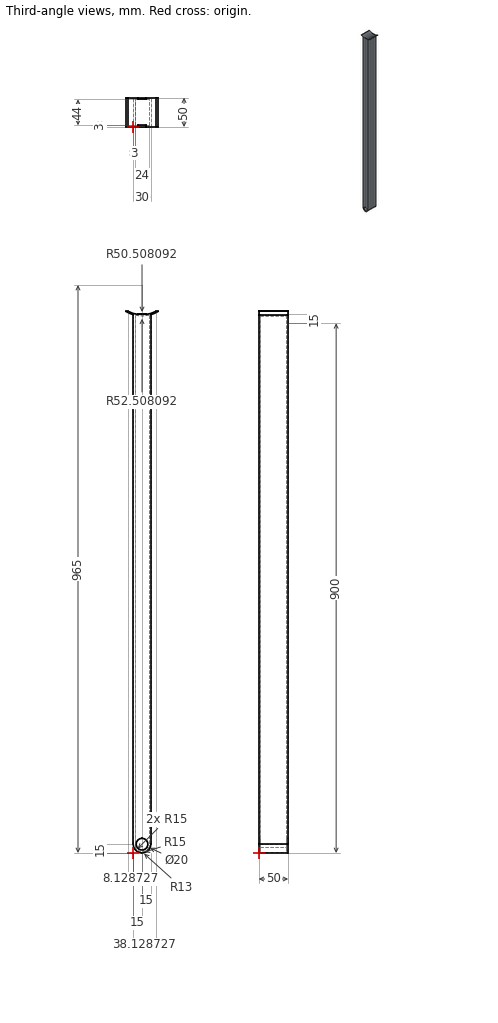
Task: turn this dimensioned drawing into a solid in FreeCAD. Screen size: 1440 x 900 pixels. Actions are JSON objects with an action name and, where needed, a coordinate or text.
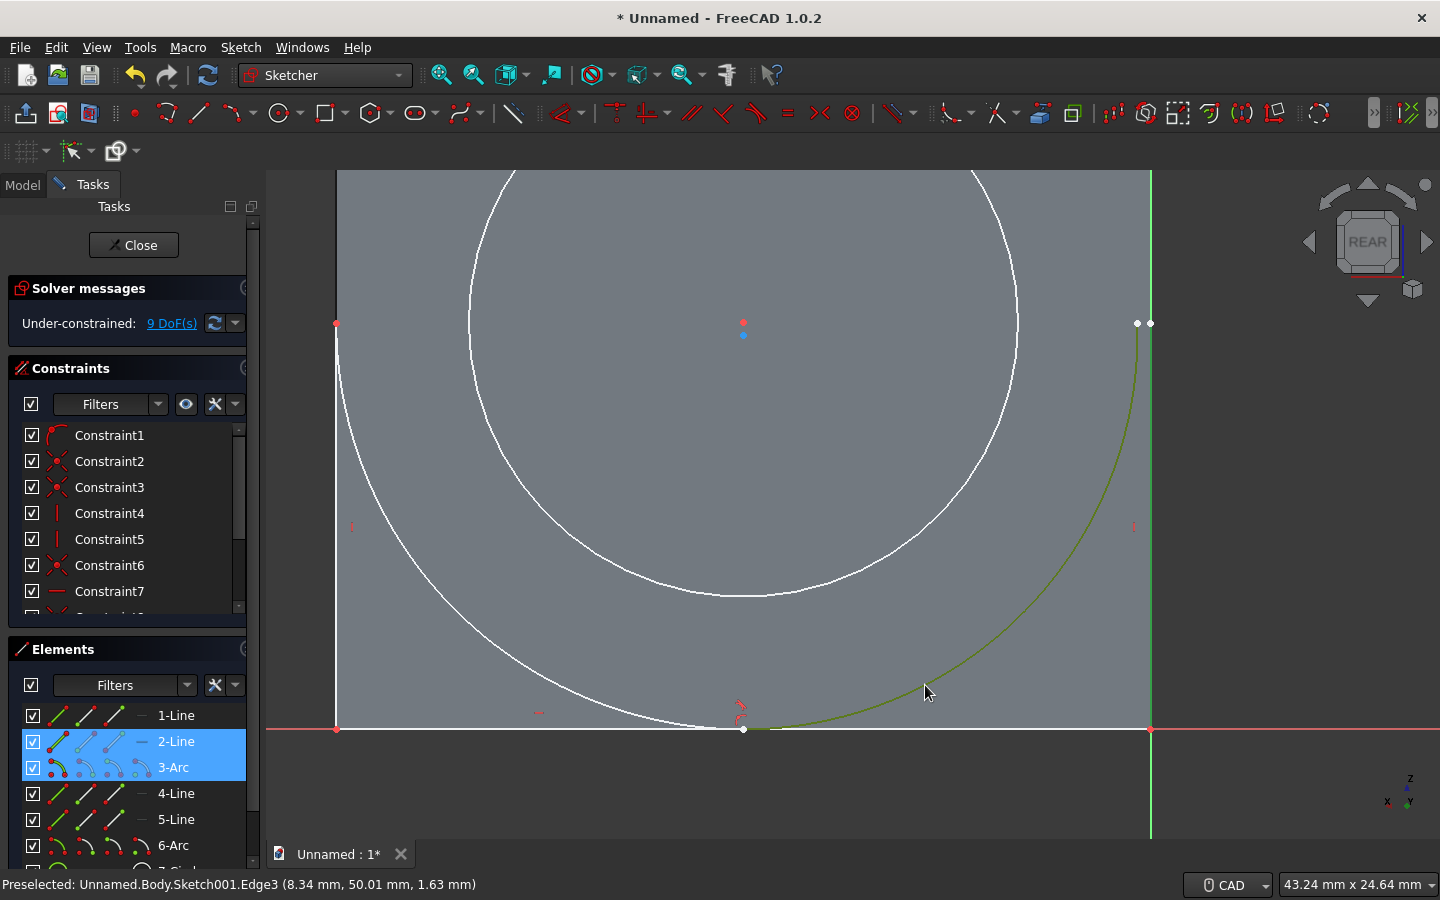
{"action": "left_click", "coordinate": [756, 114]}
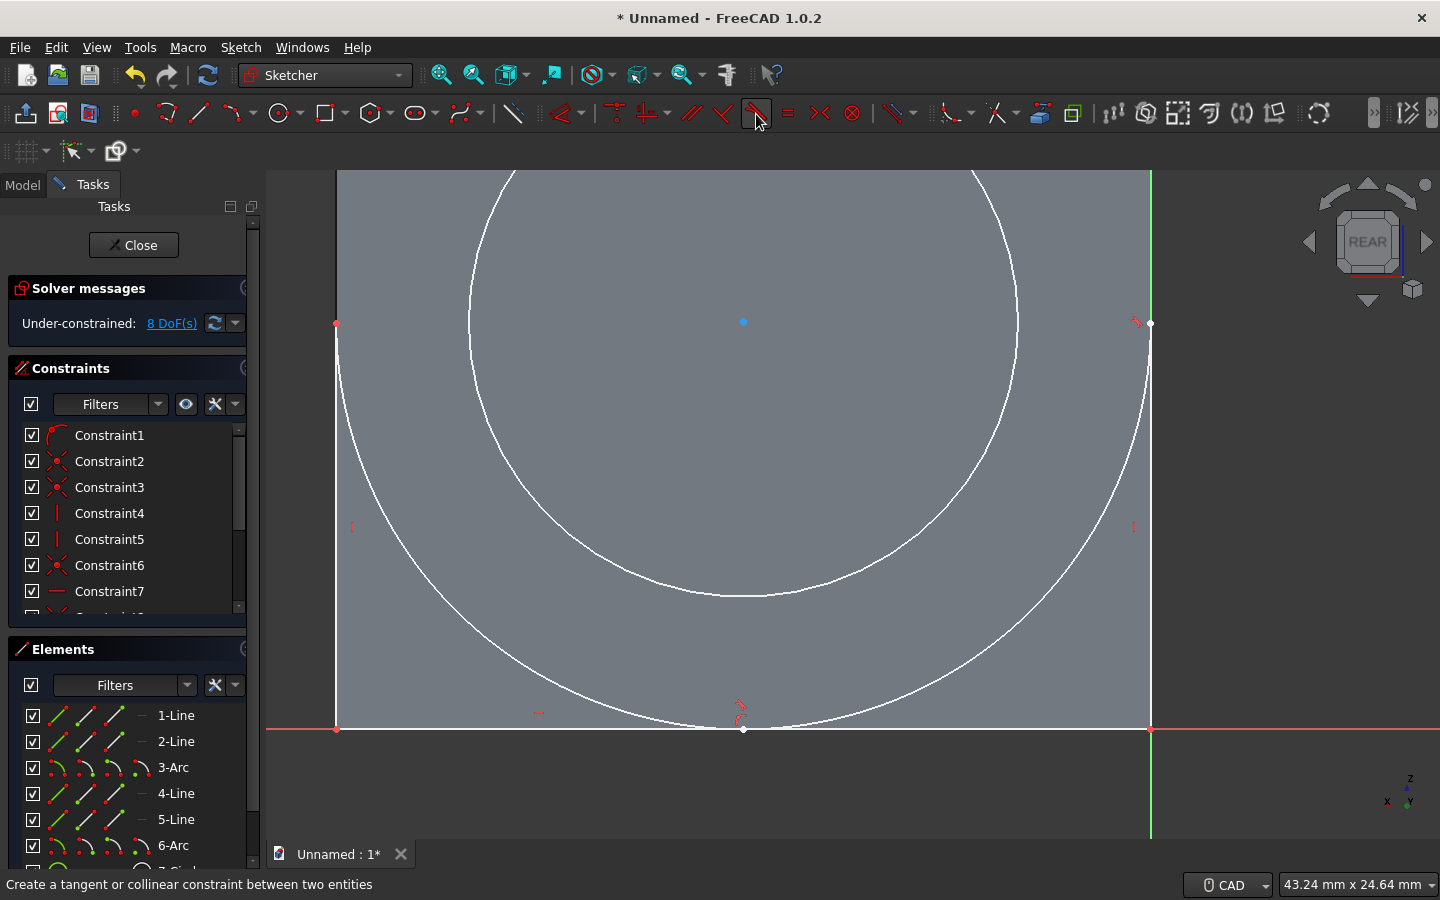
{"action": "left_click", "coordinate": [928, 685]}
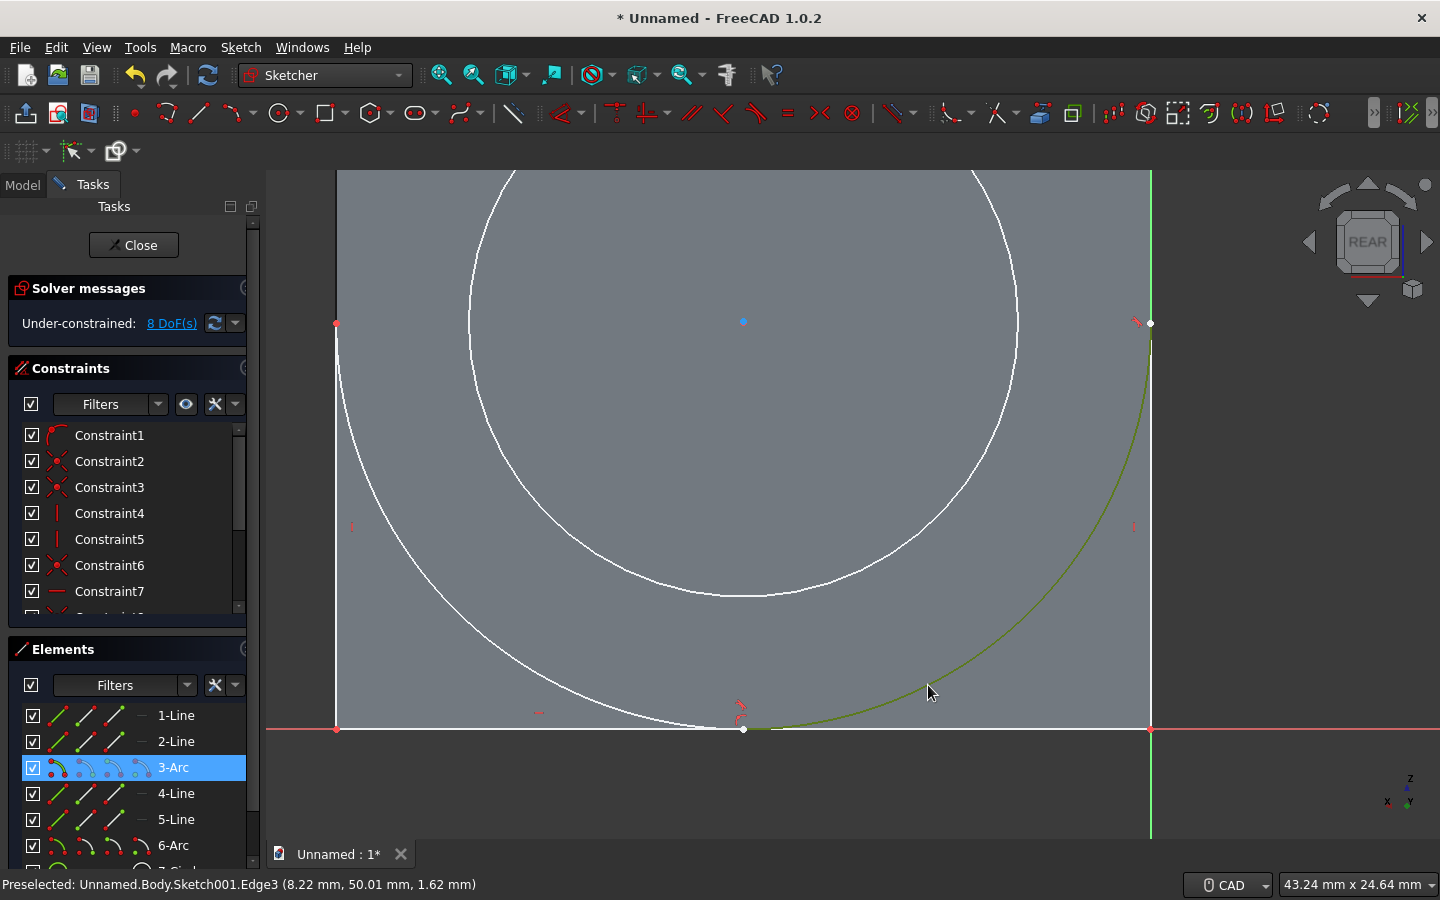
{"action": "left_click", "coordinate": [458, 729]}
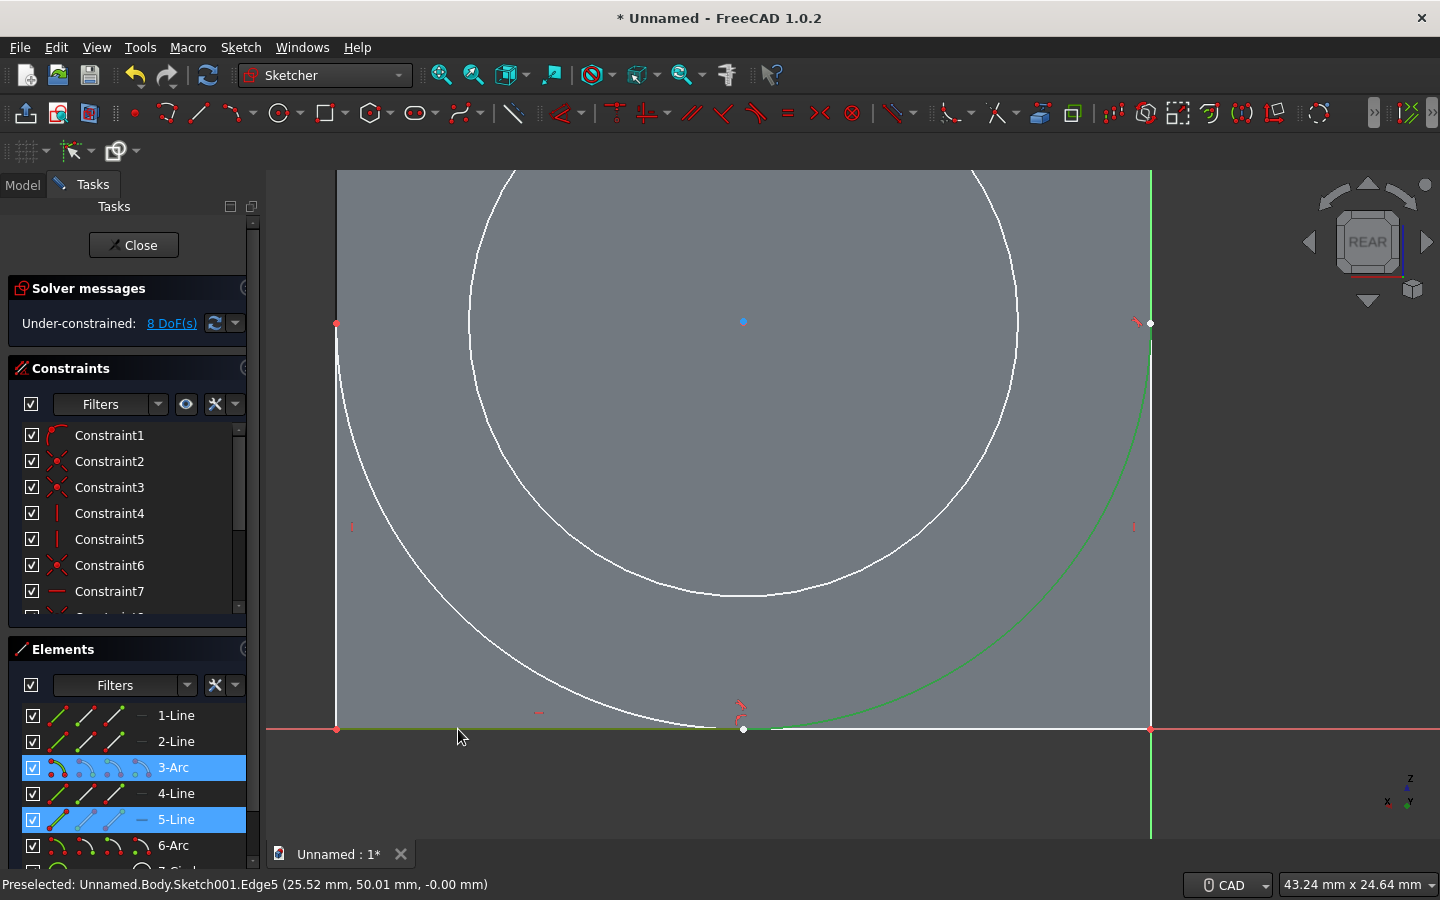
{"action": "left_click", "coordinate": [756, 114]}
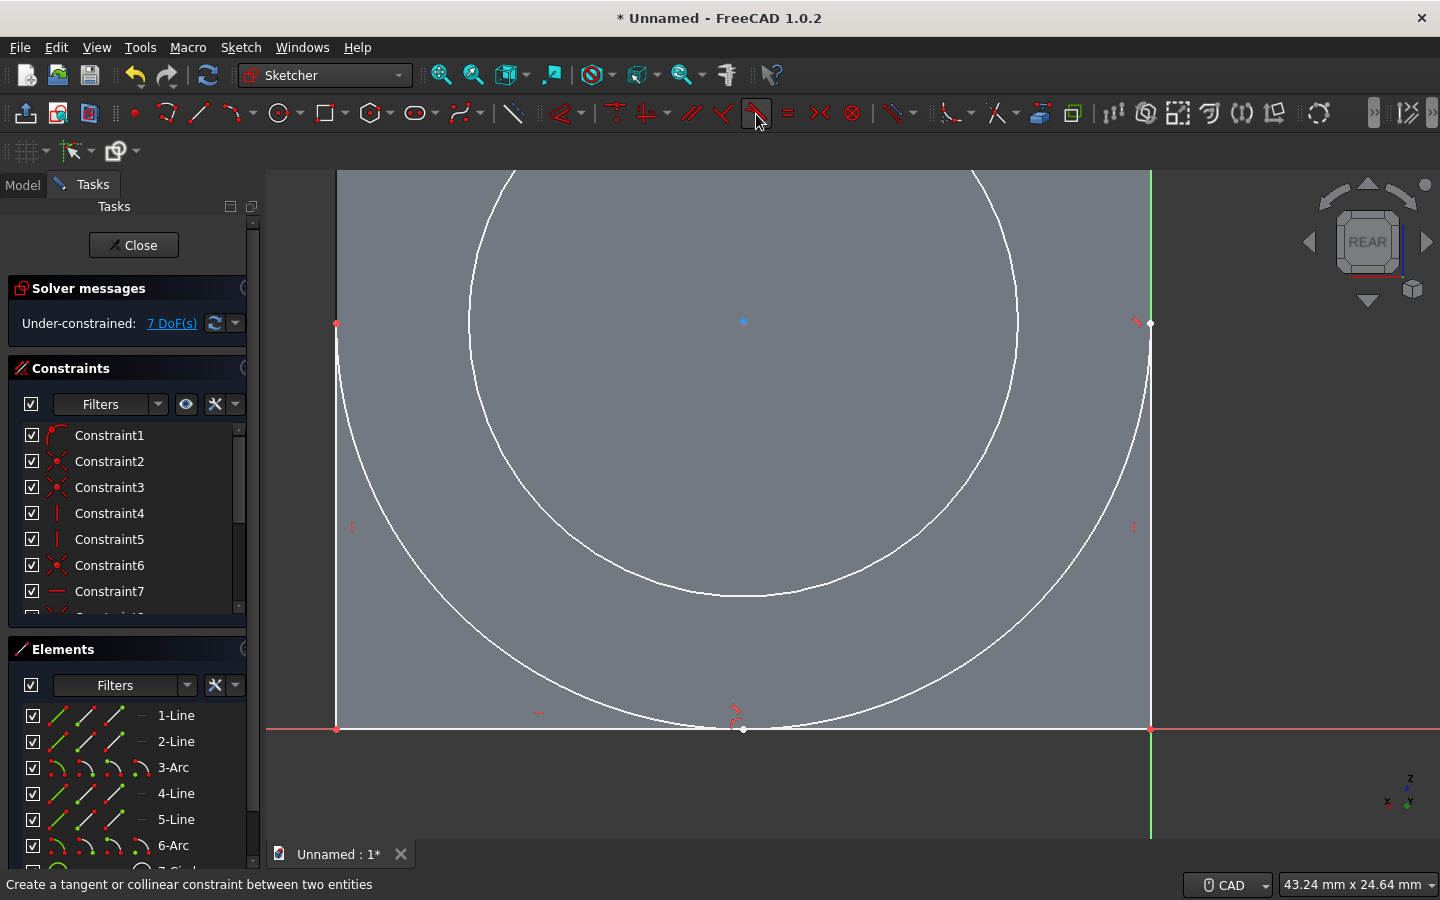
{"action": "left_click", "coordinate": [336, 445]}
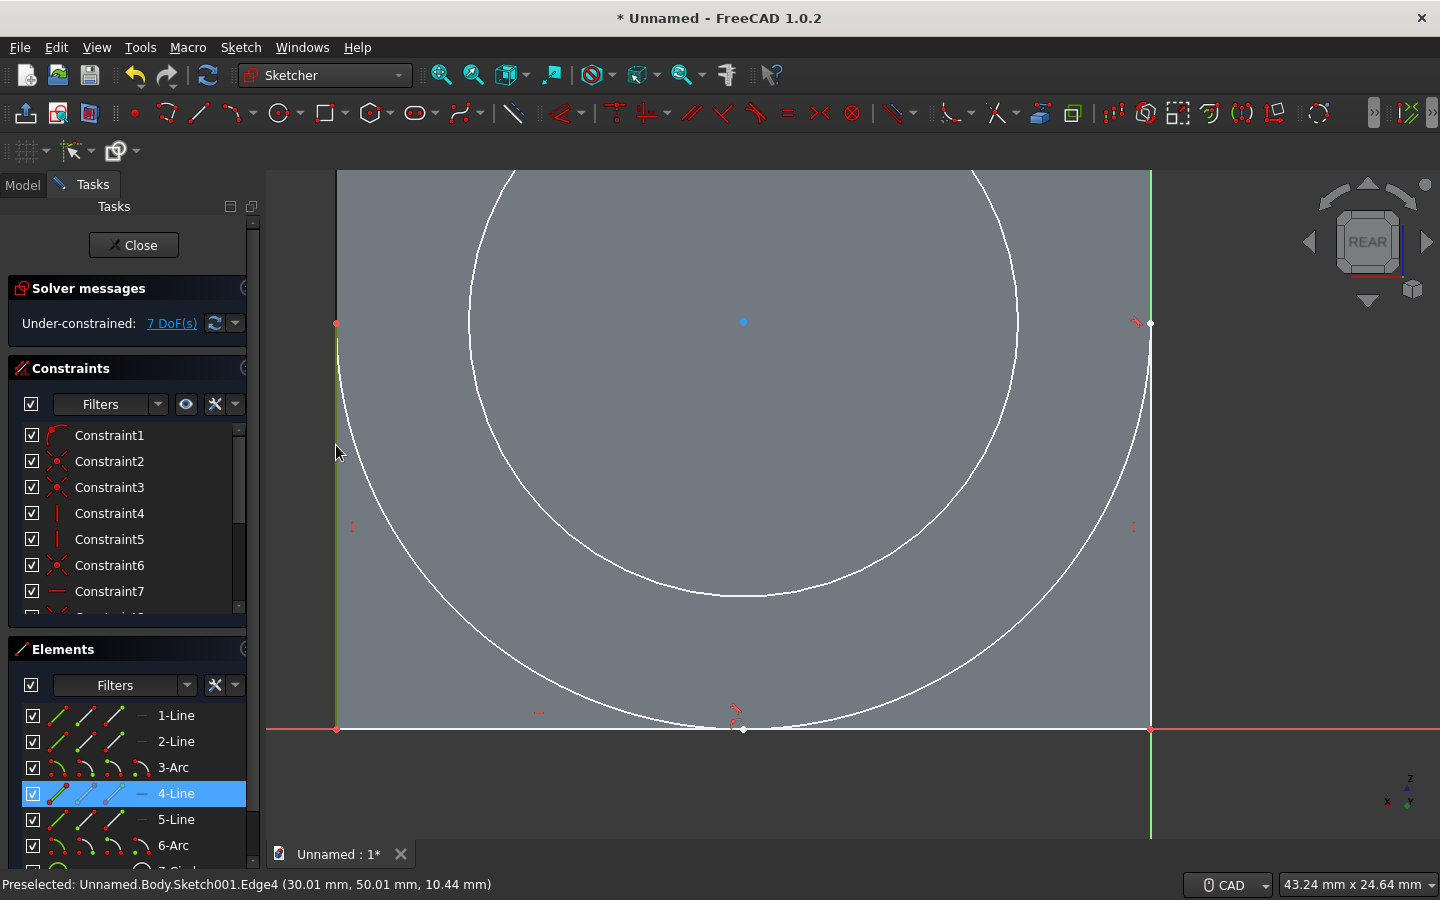
{"action": "left_click", "coordinate": [381, 508]}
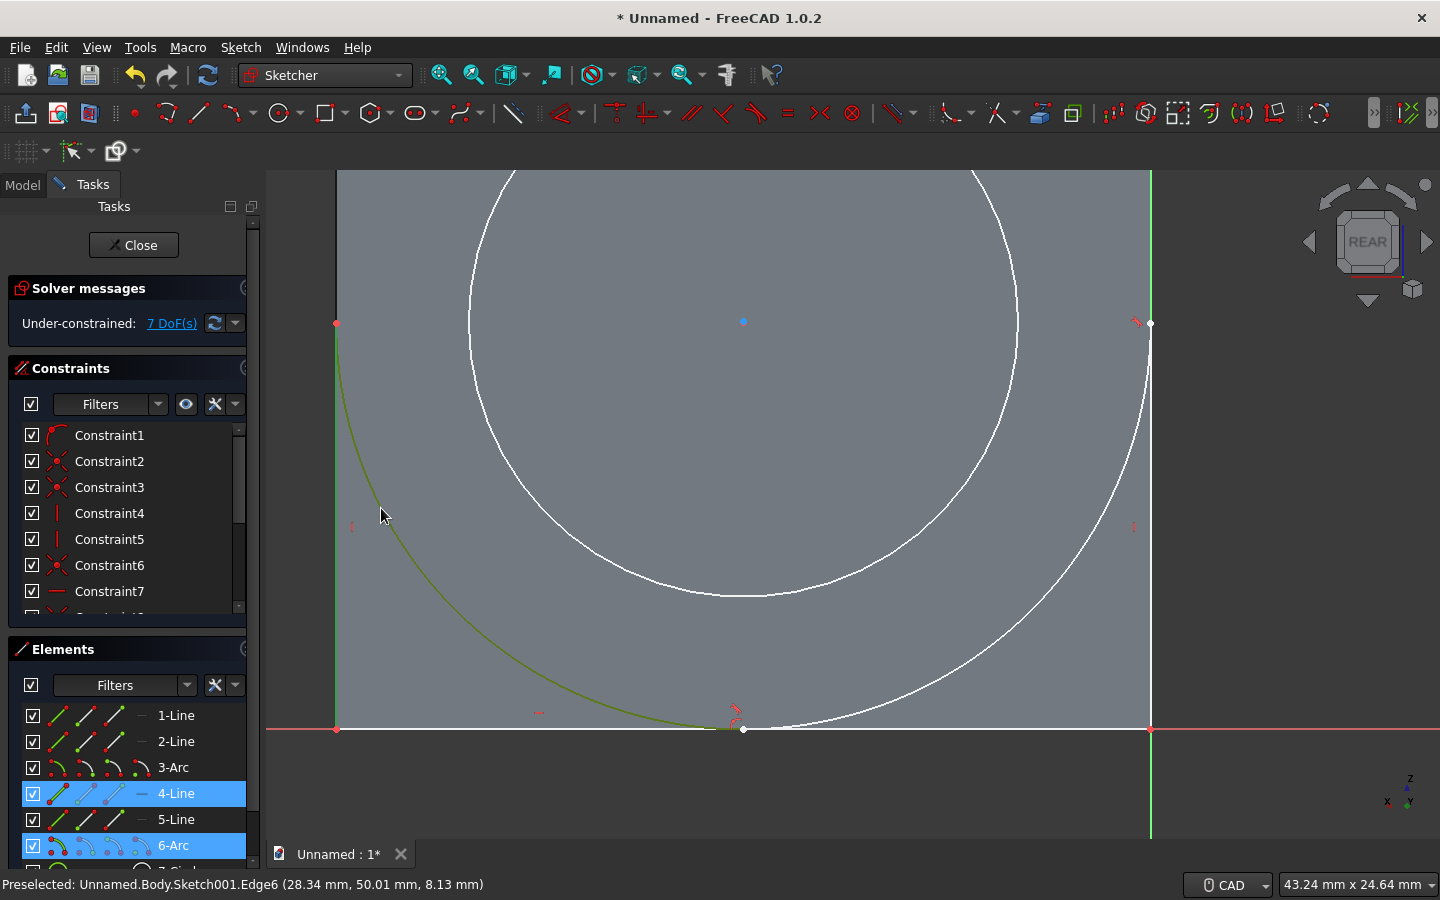
{"action": "left_click", "coordinate": [756, 114]}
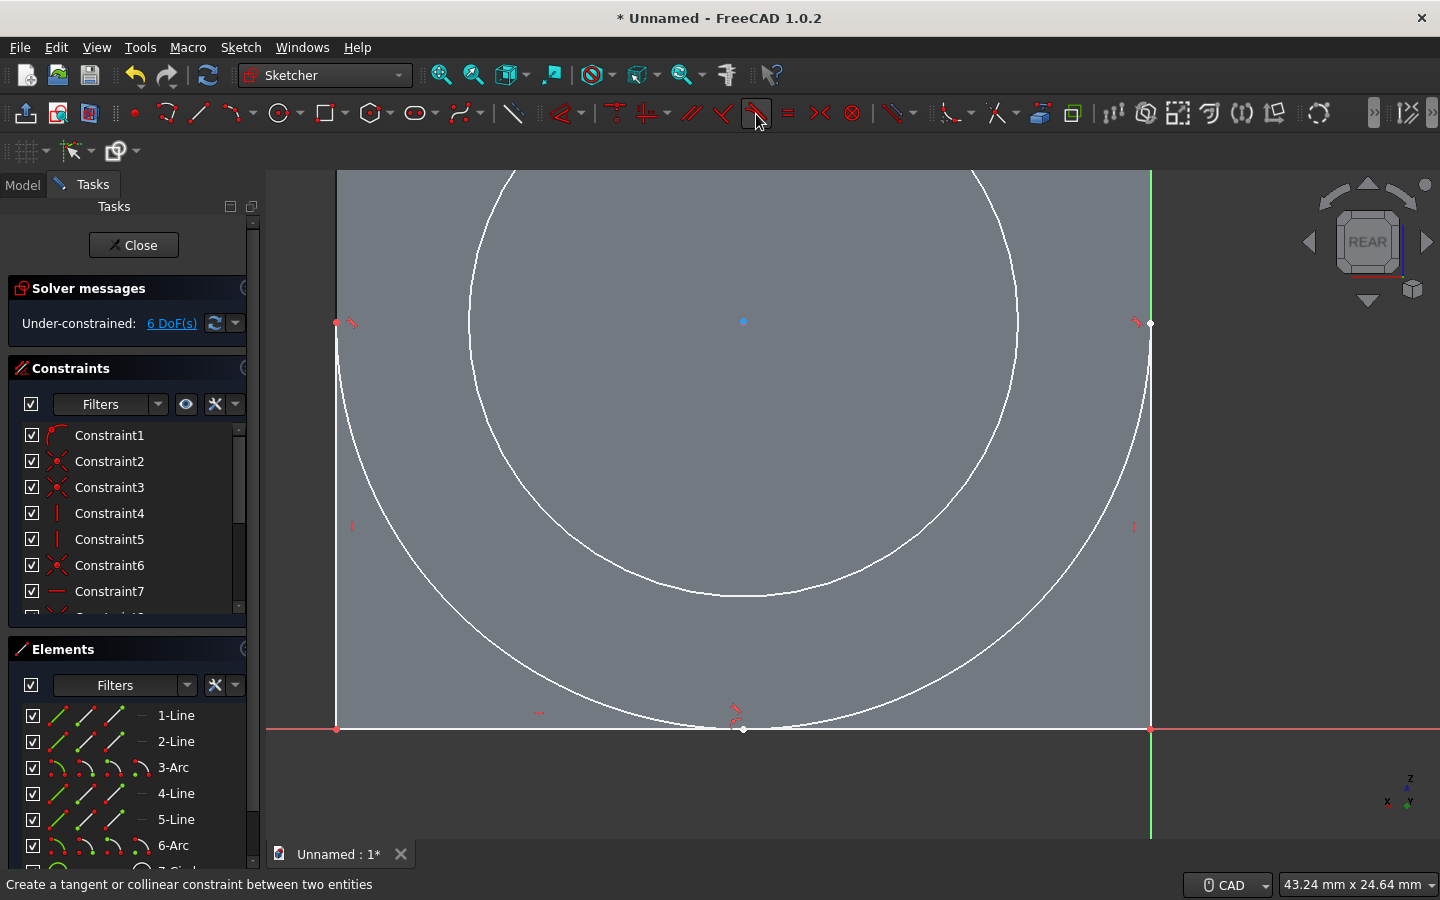
{"action": "left_click", "coordinate": [928, 685]}